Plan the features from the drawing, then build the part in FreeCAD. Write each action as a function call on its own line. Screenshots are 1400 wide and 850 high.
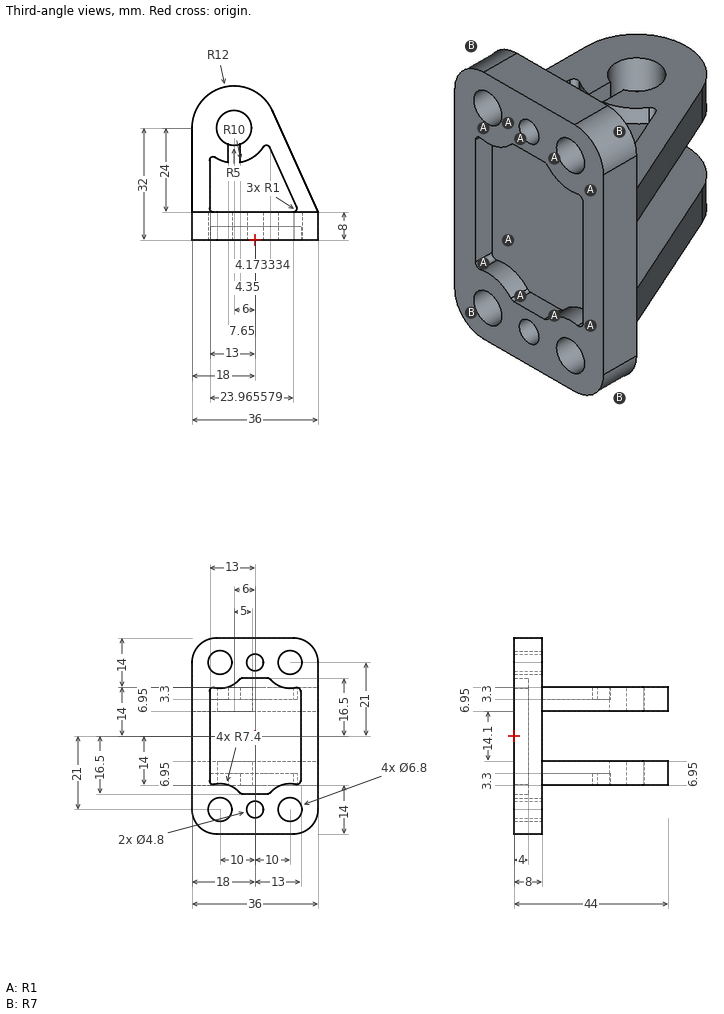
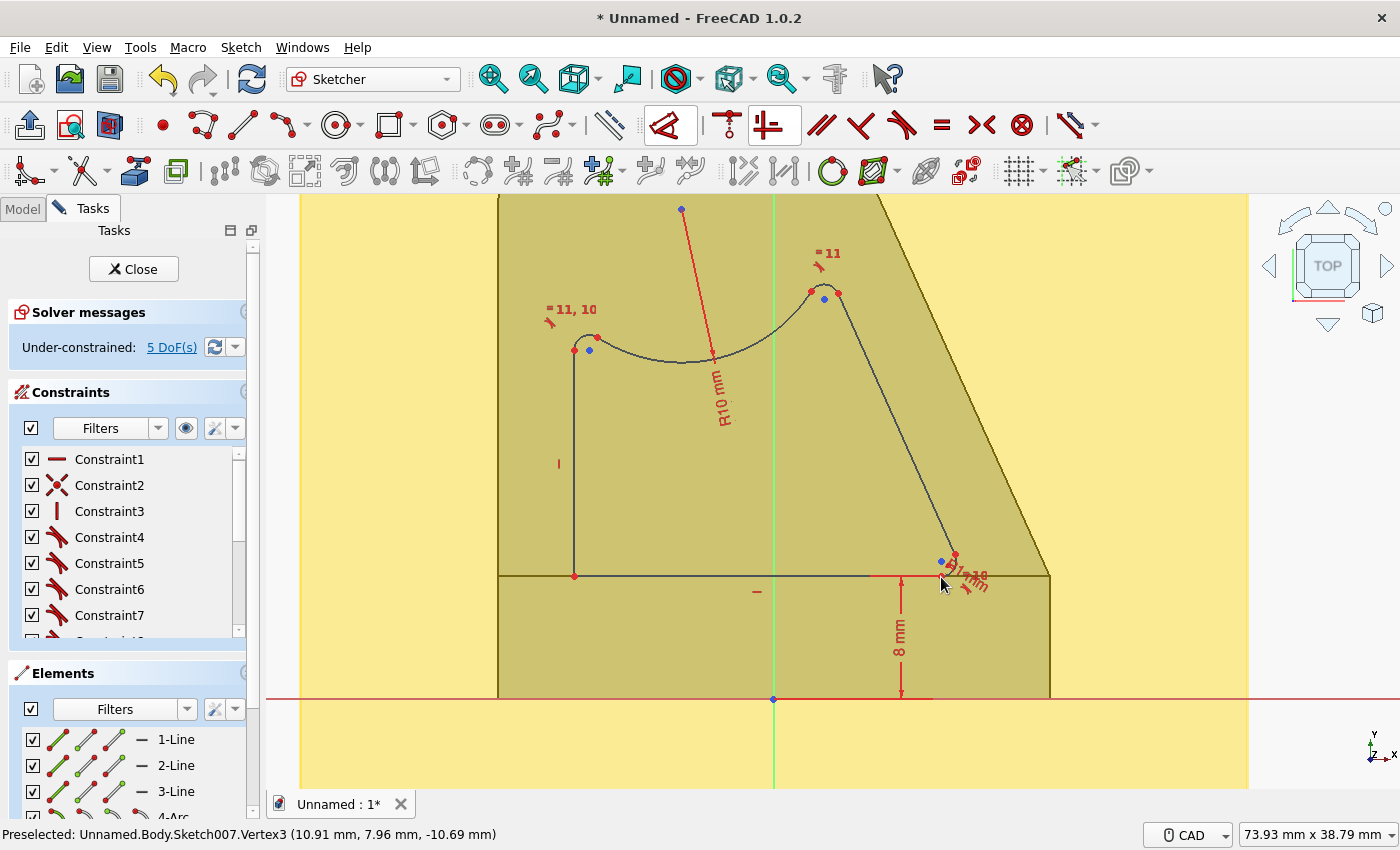
scroll(762, 660, down, 1)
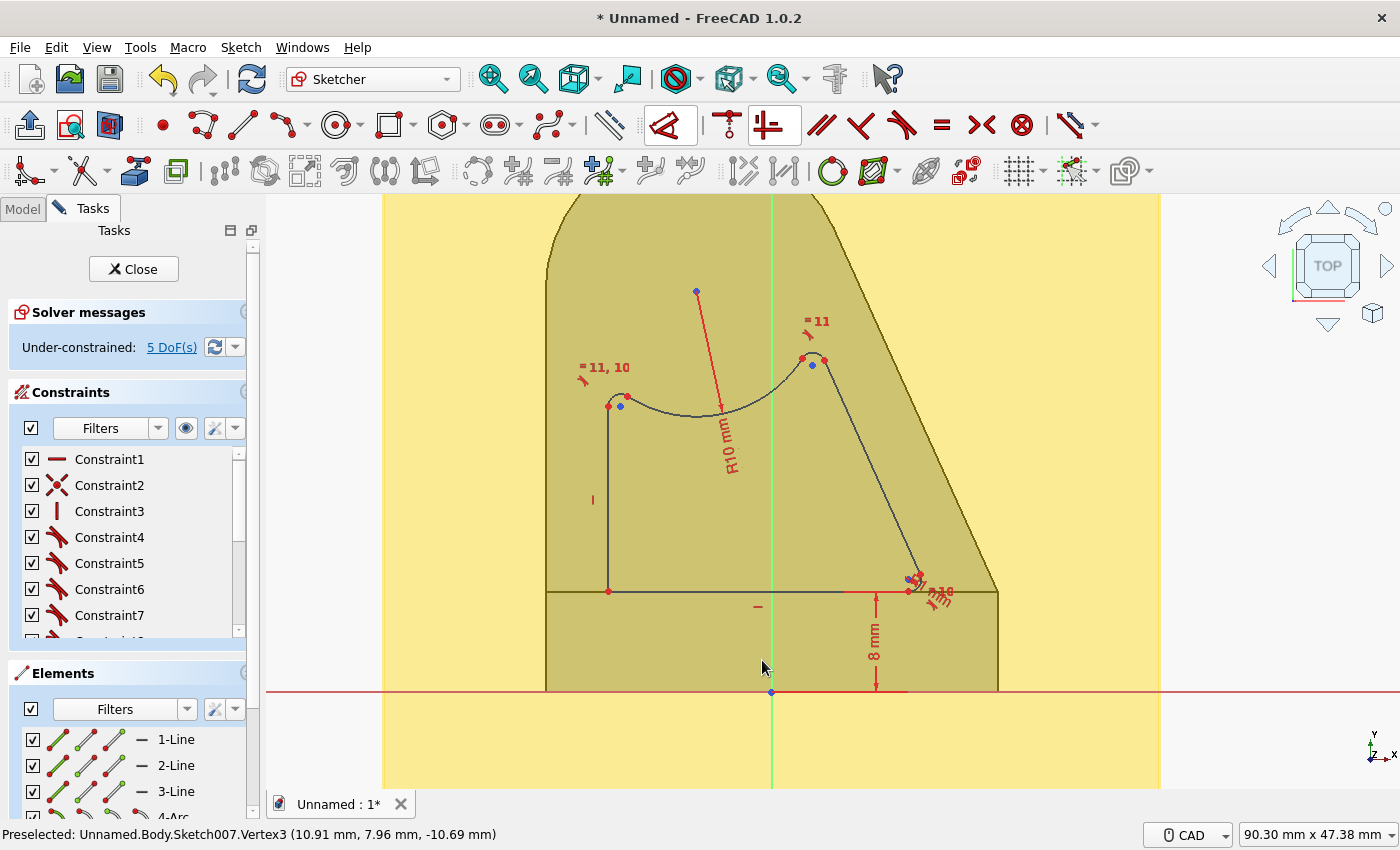
click(696, 291)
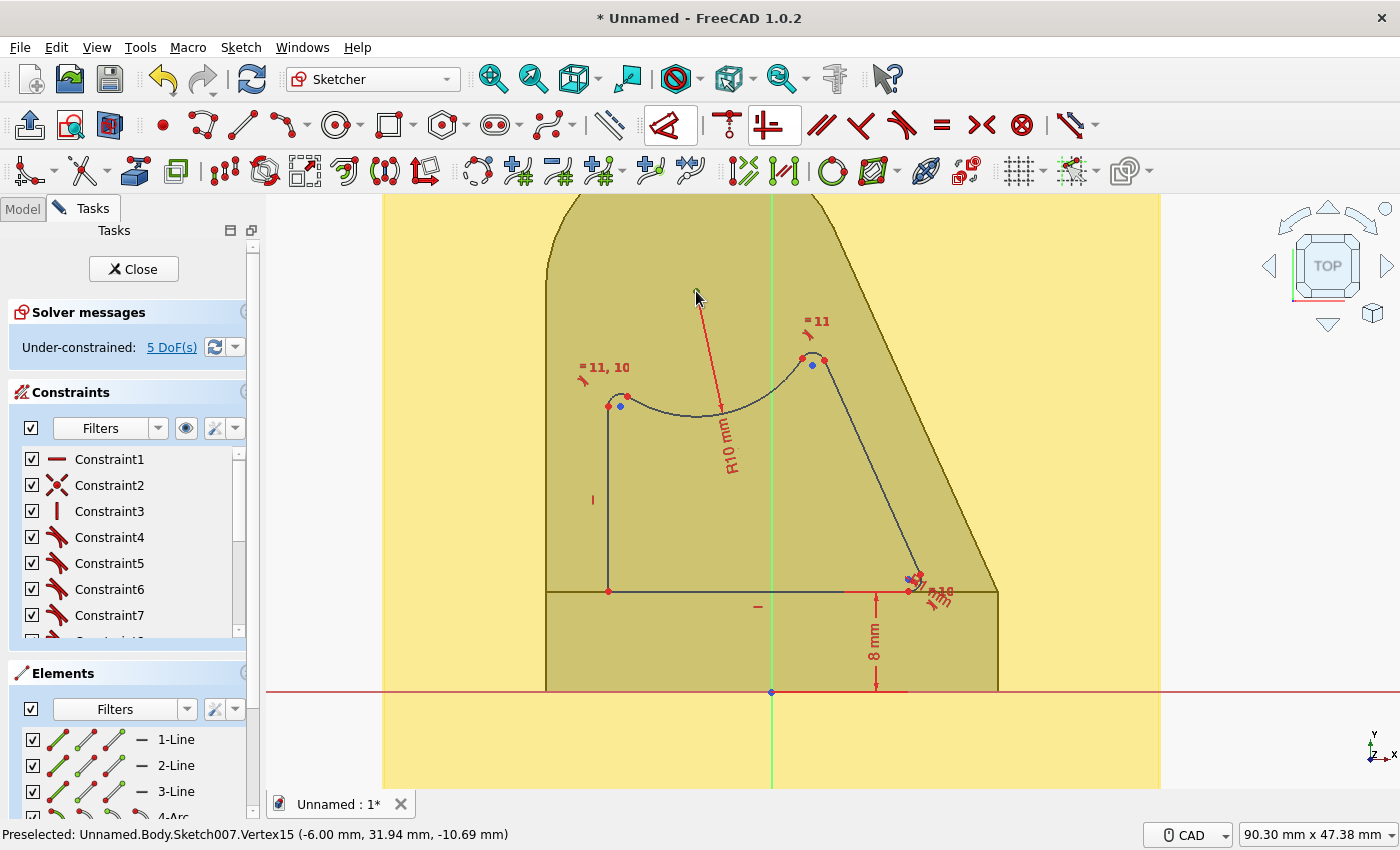
key(l)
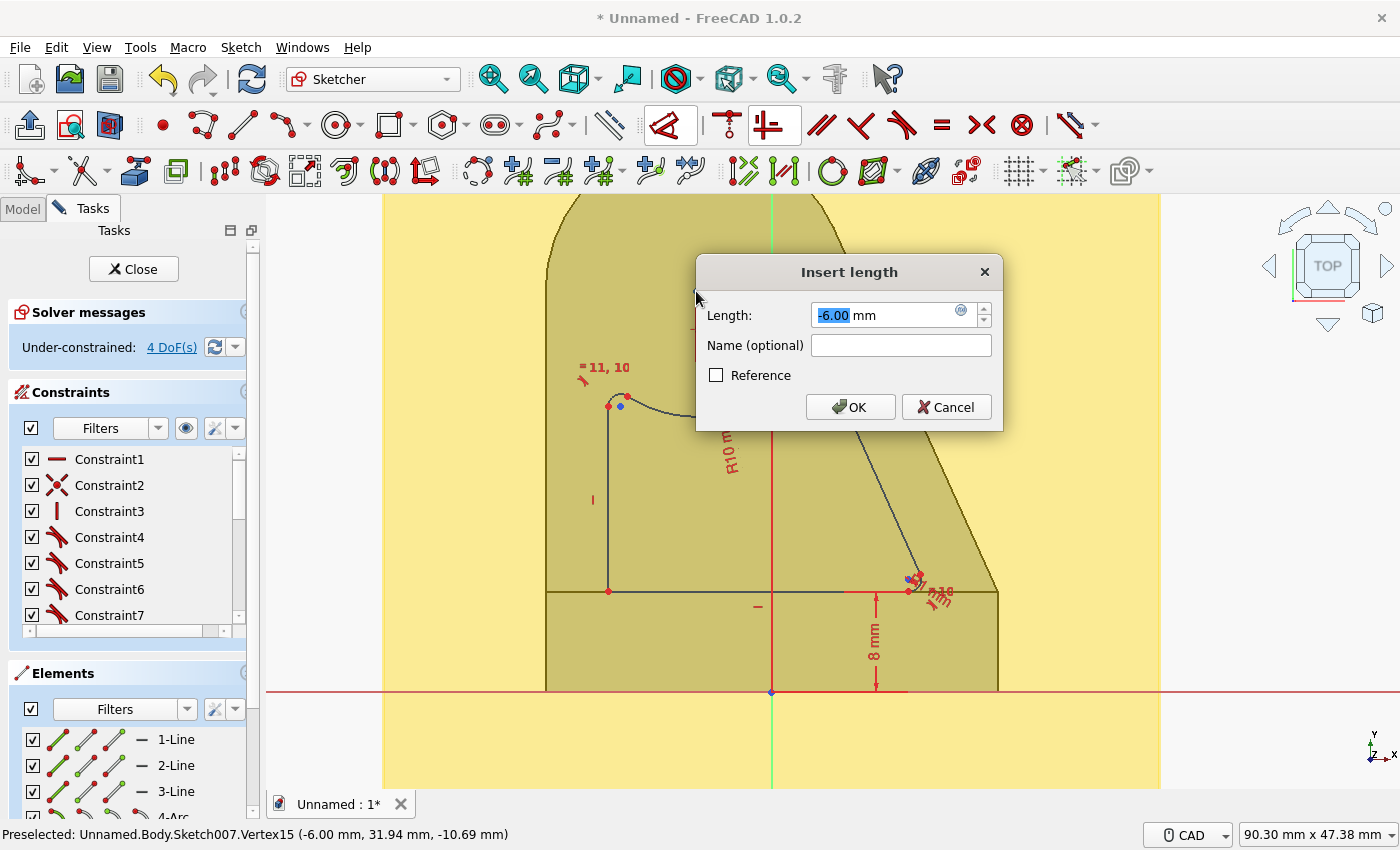
text(-6)
key(Return)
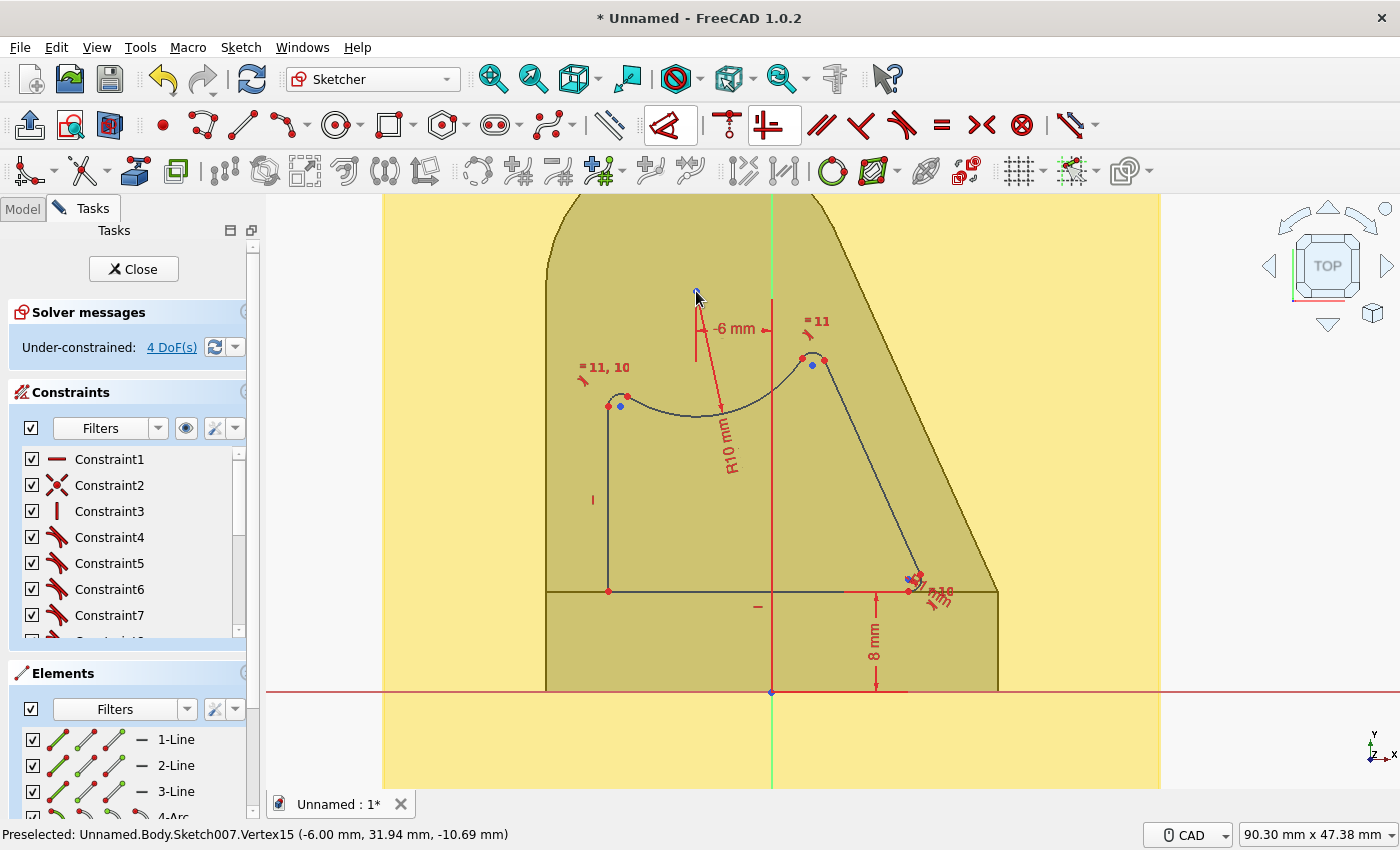
click(608, 592)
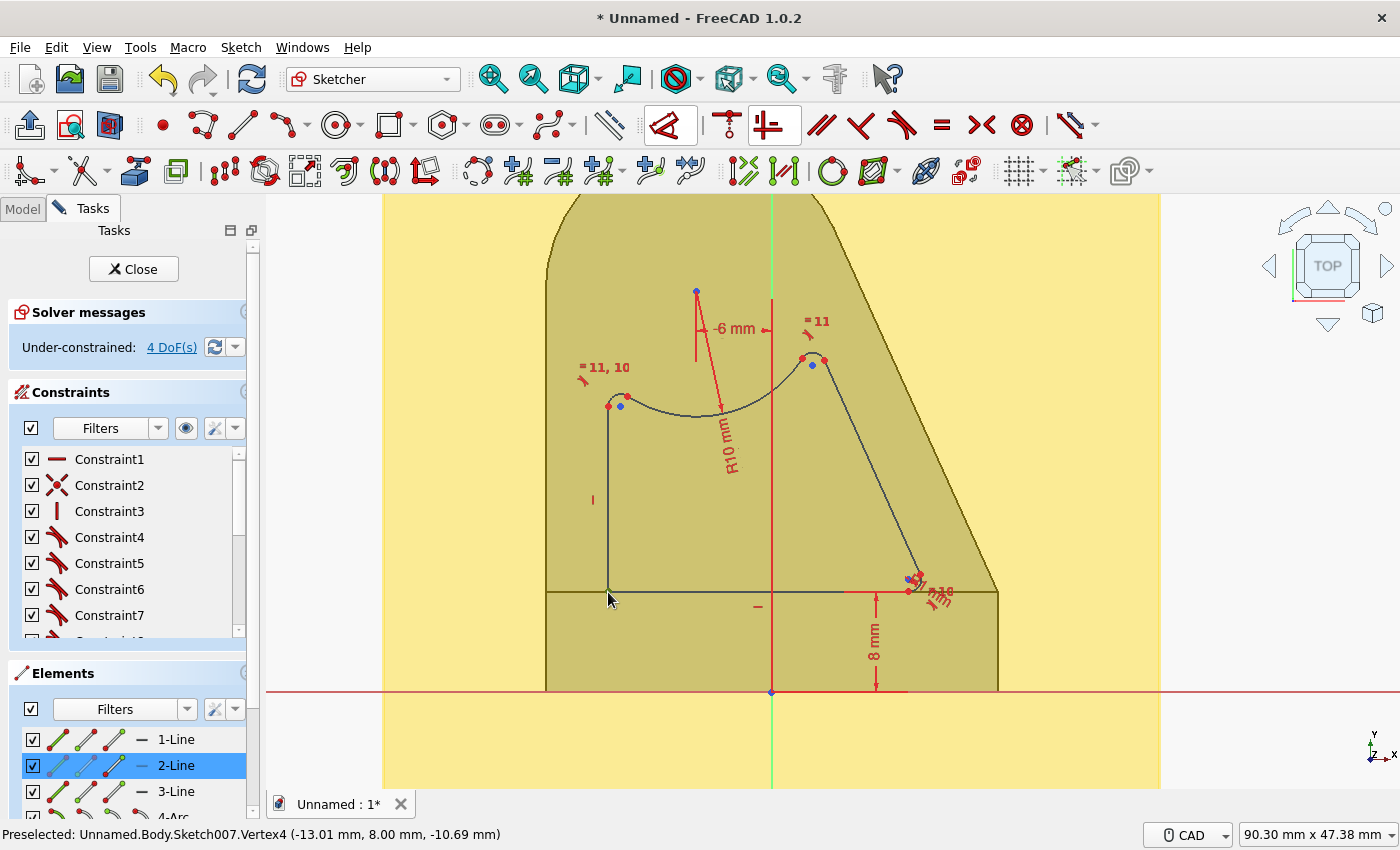
key(l)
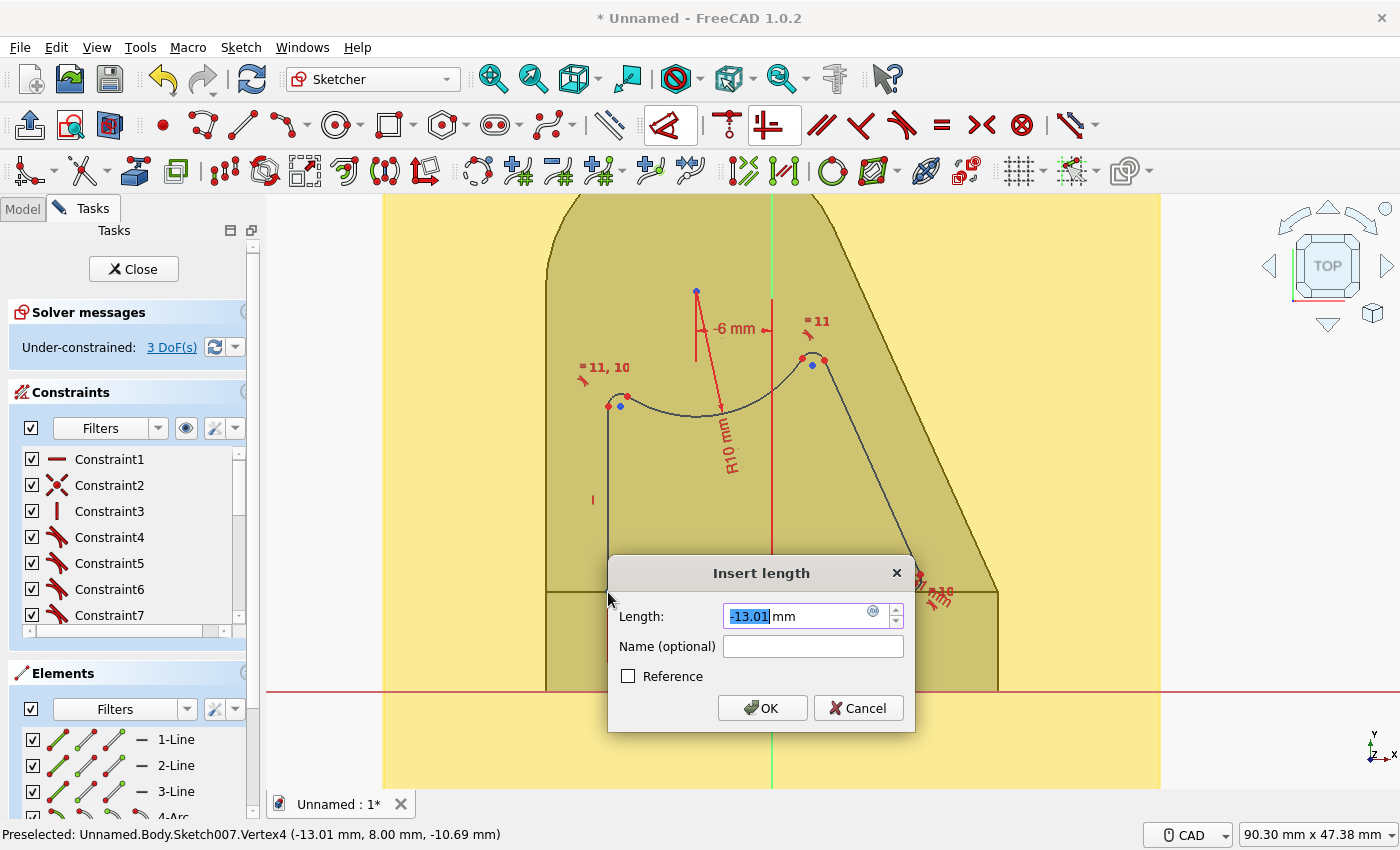
text(-13)
key(Return)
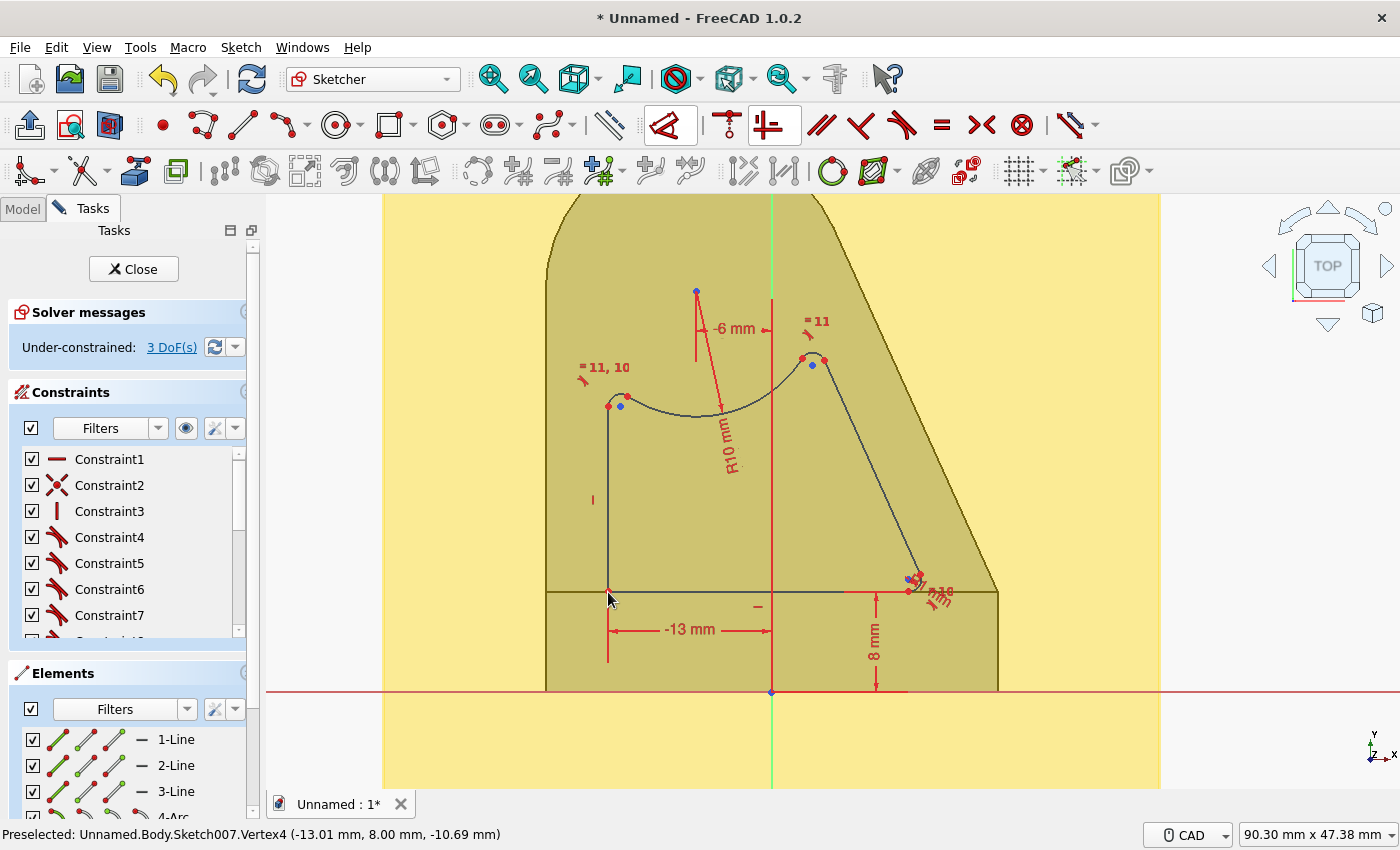
click(696, 291)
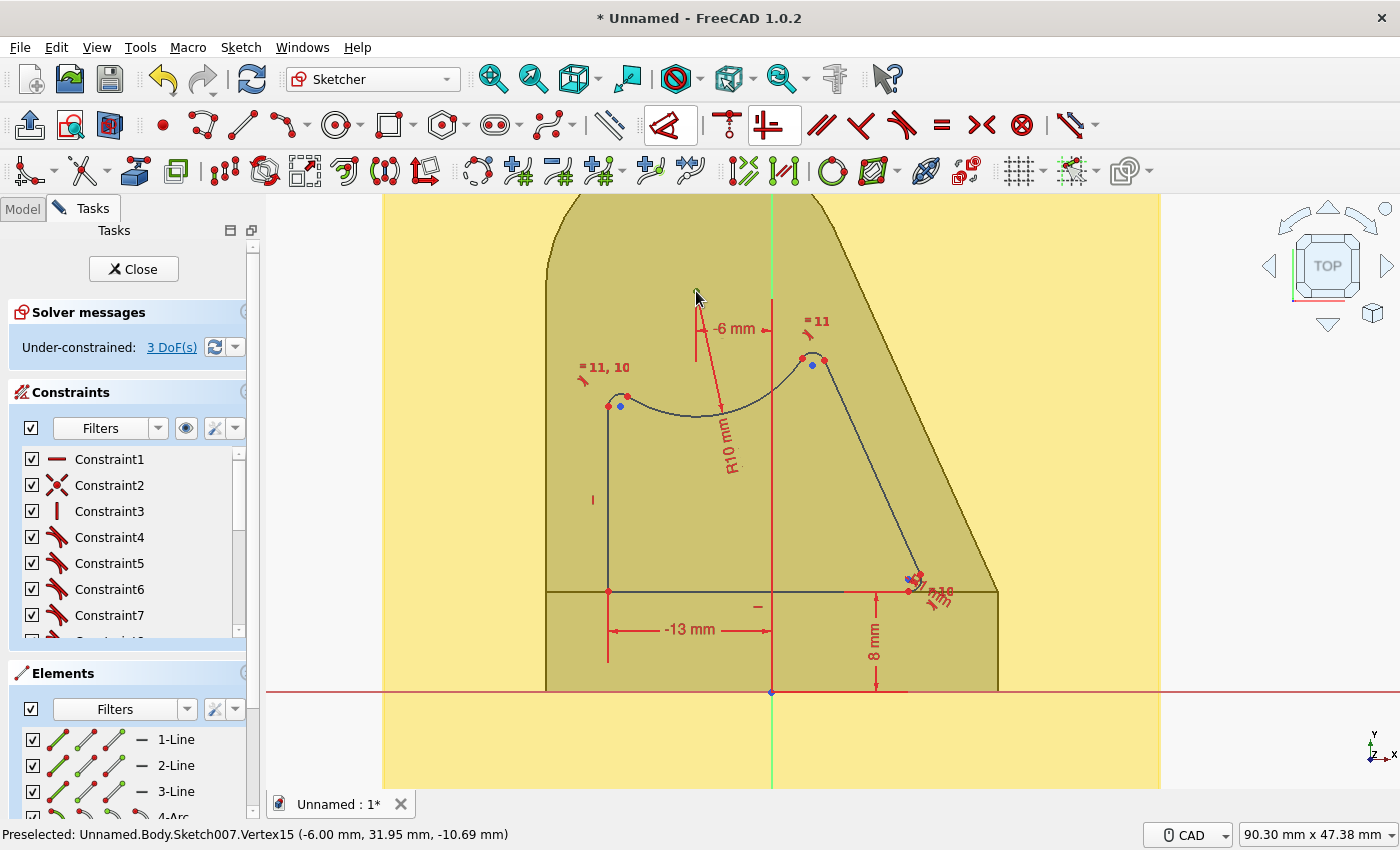
click(692, 126)